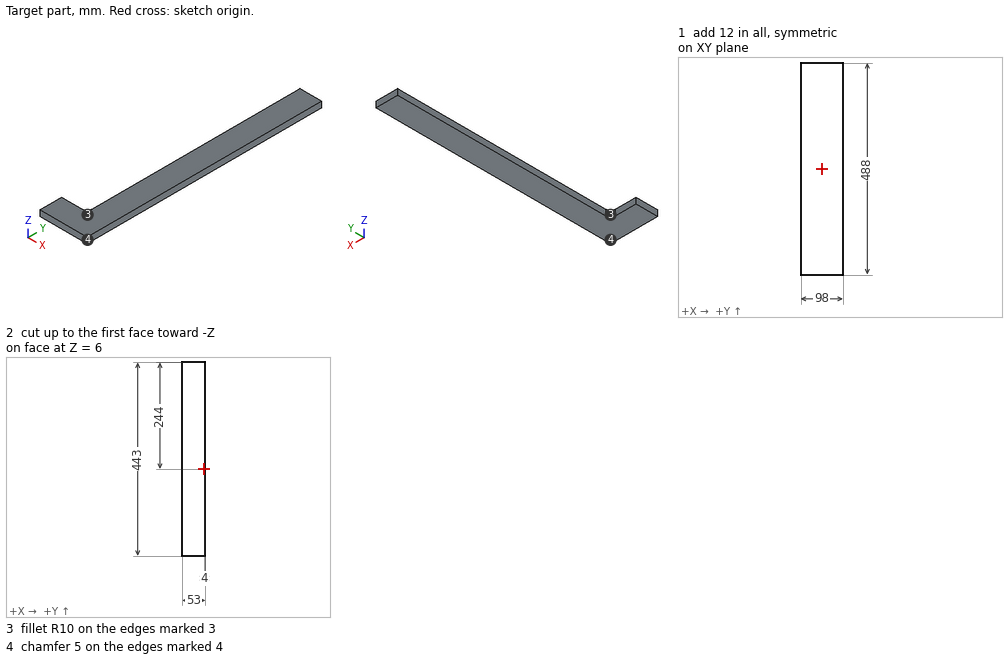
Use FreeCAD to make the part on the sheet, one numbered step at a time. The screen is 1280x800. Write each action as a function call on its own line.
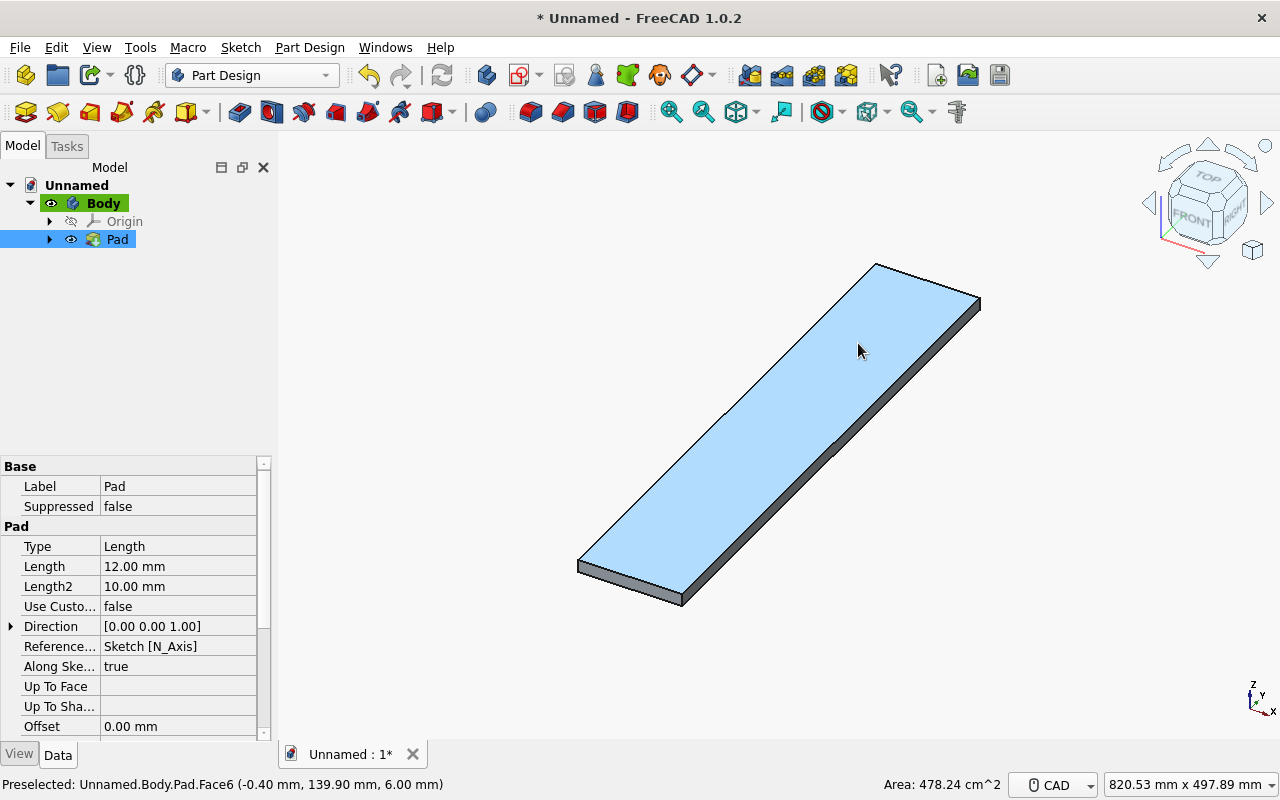
click(520, 76)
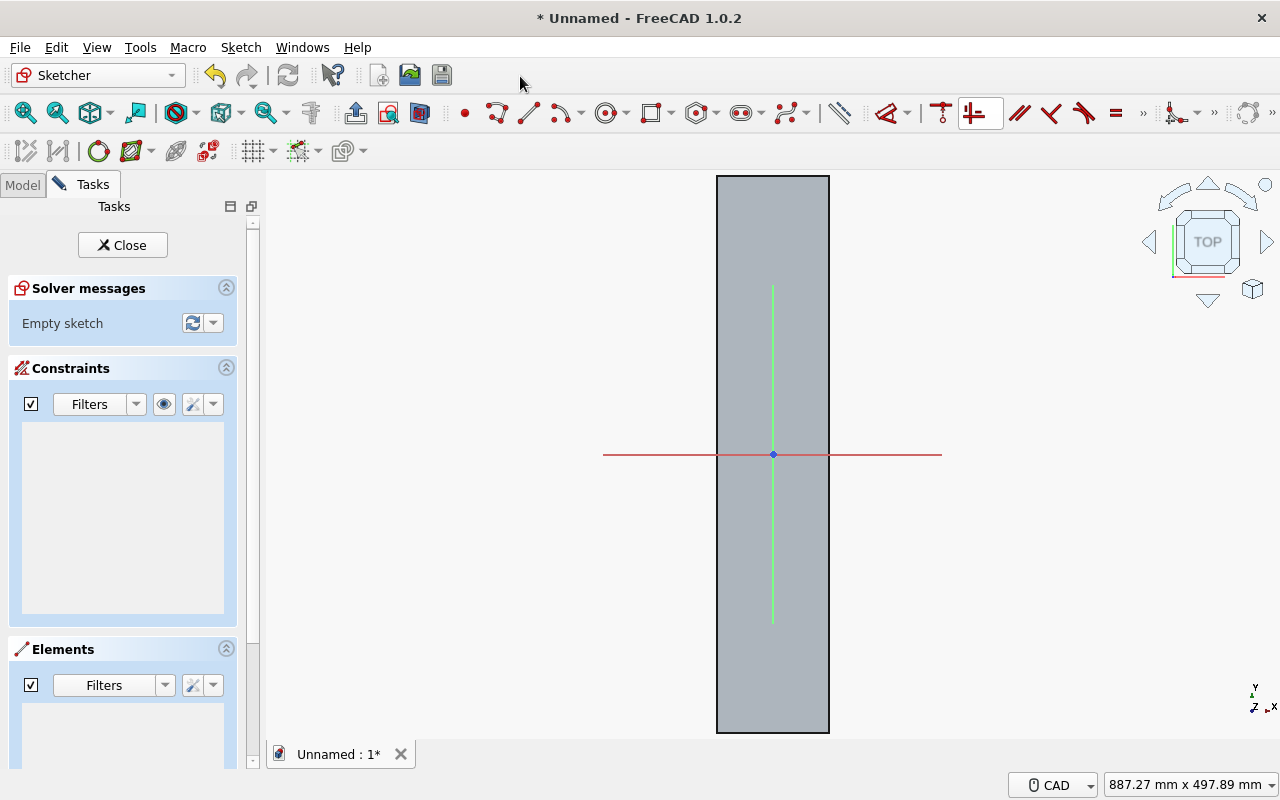
scroll(618, 507, down, 2)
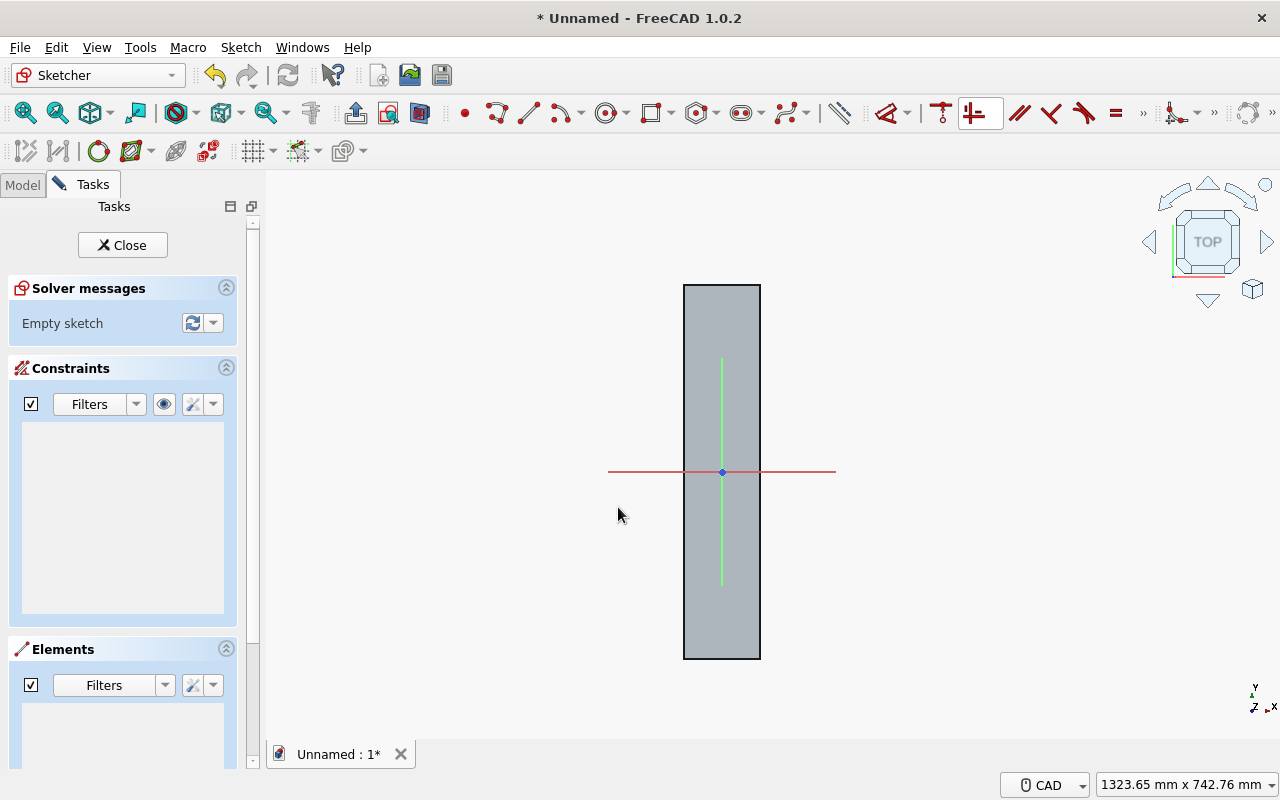
key(g)
key(r)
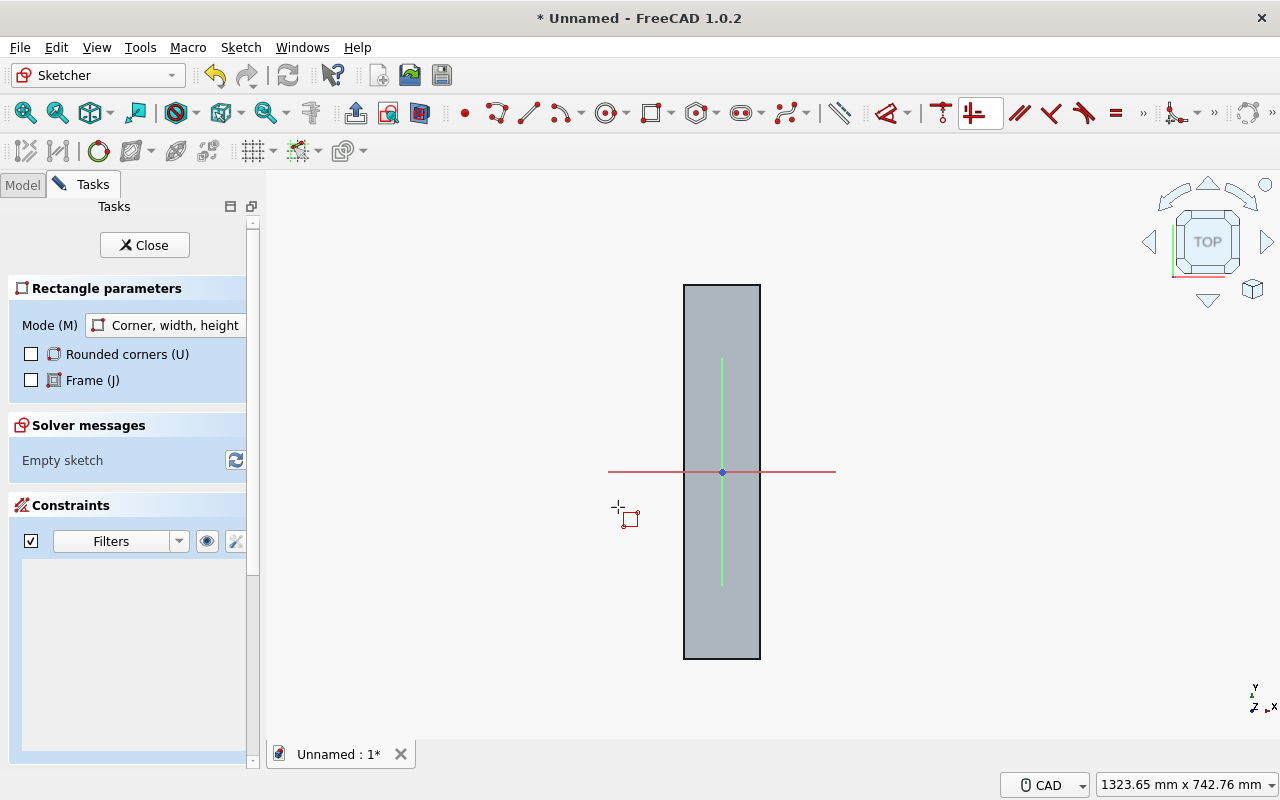
click(684, 285)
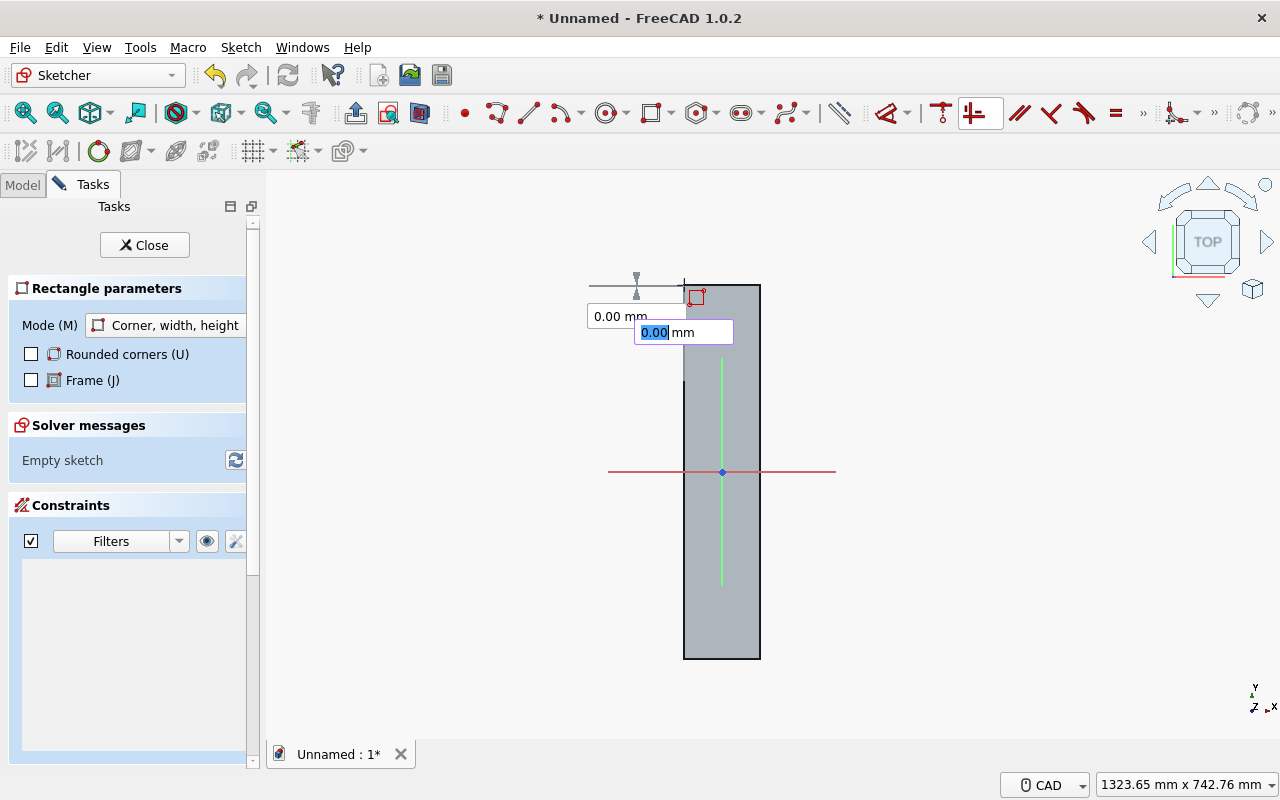
scroll(725, 624, up, 9)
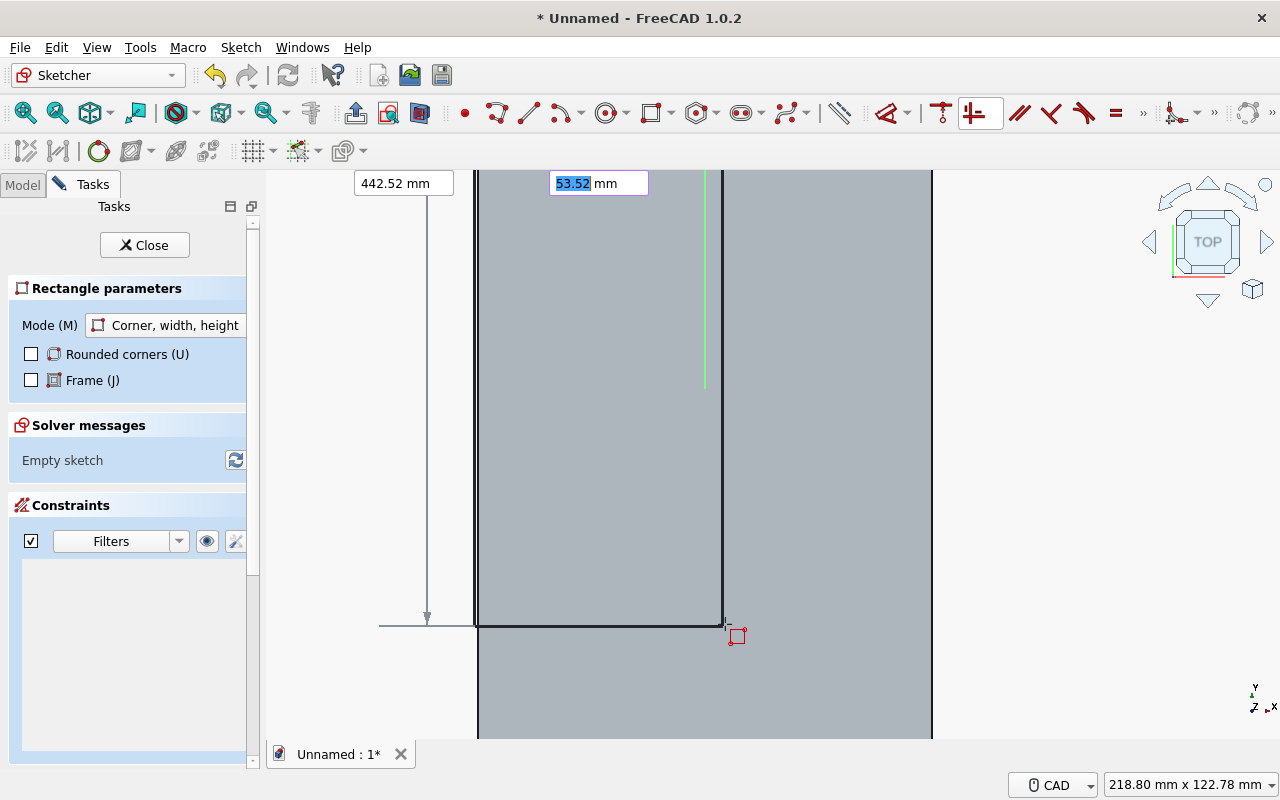
click(723, 623)
key(Escape)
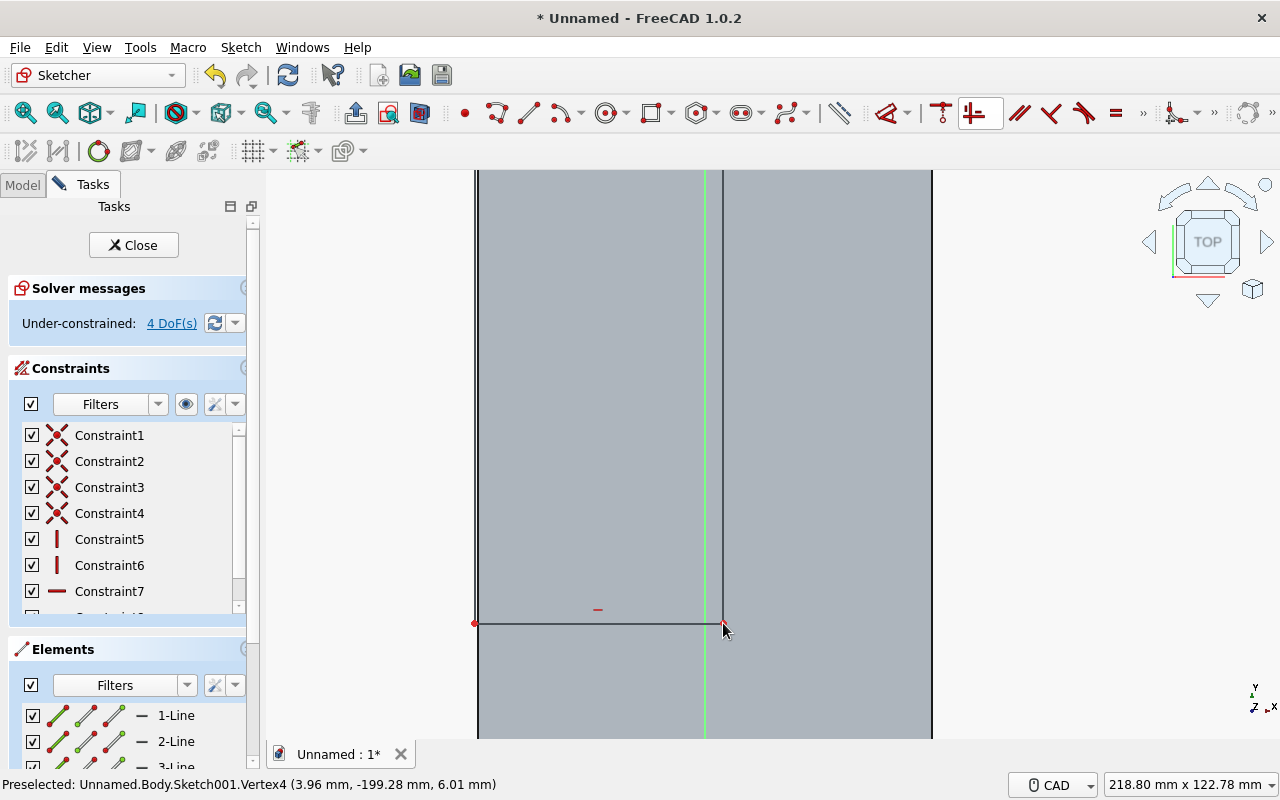
scroll(725, 624, down, 9)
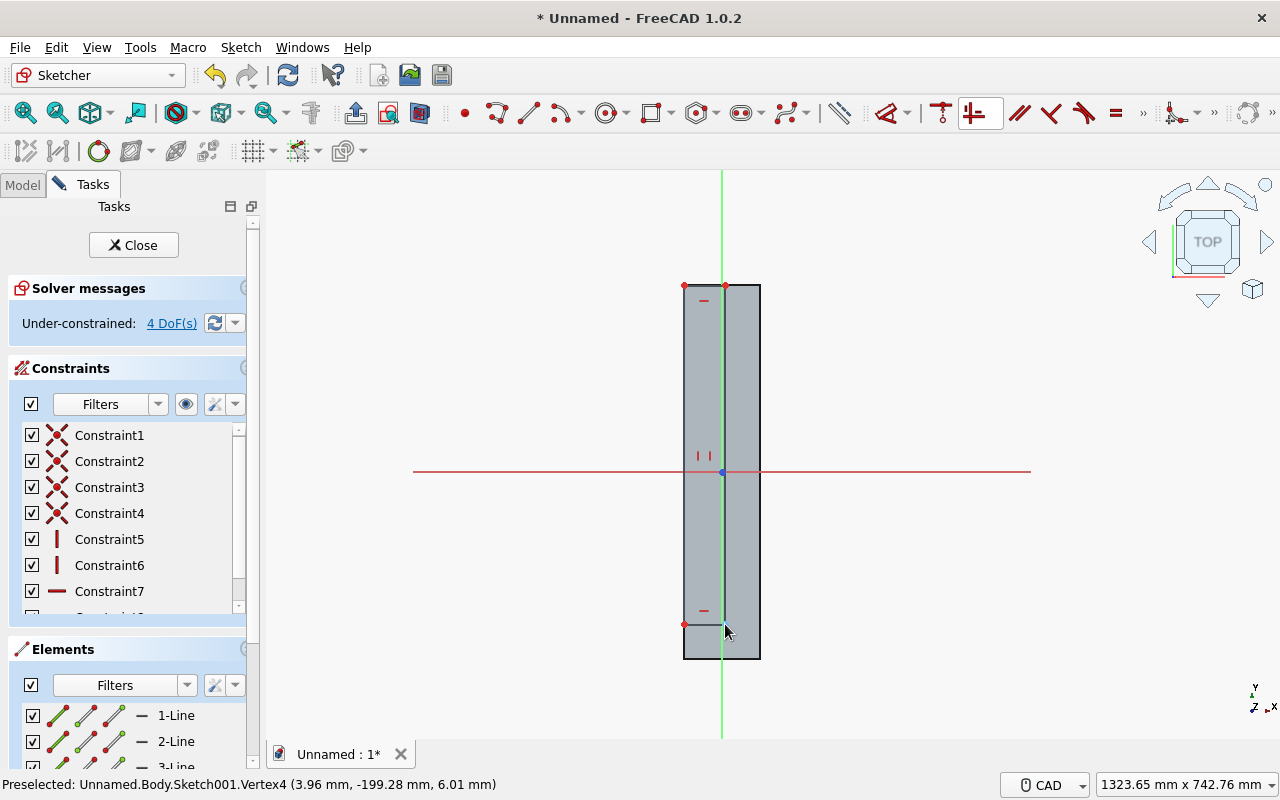
click(696, 625)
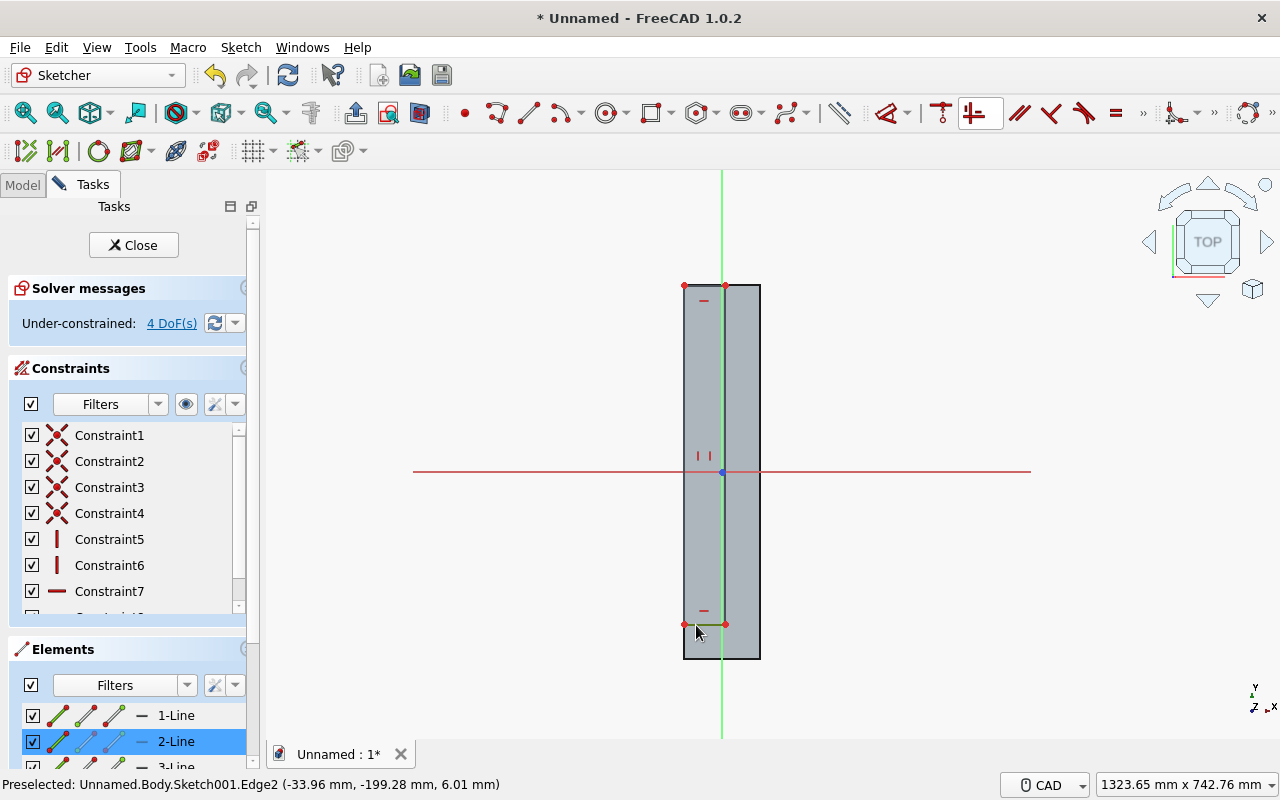
key(l)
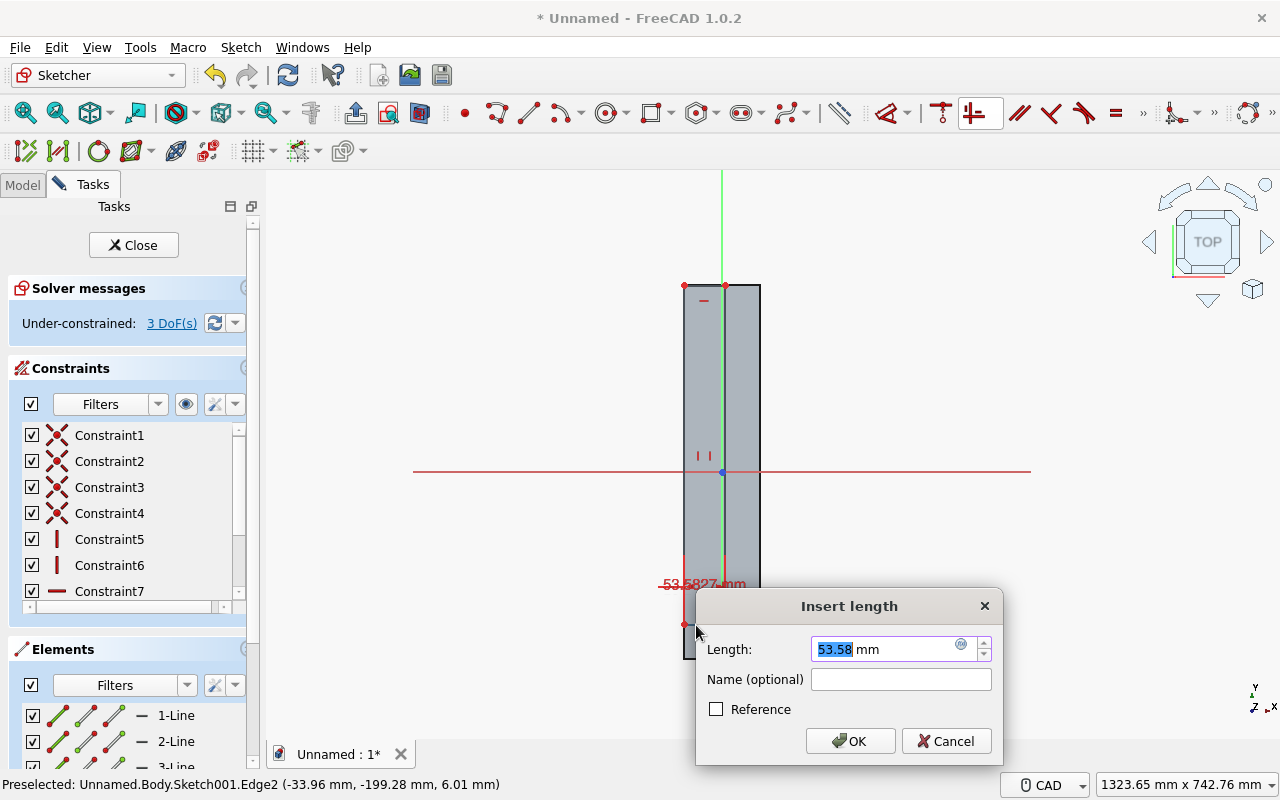
text(53)
key(Return)